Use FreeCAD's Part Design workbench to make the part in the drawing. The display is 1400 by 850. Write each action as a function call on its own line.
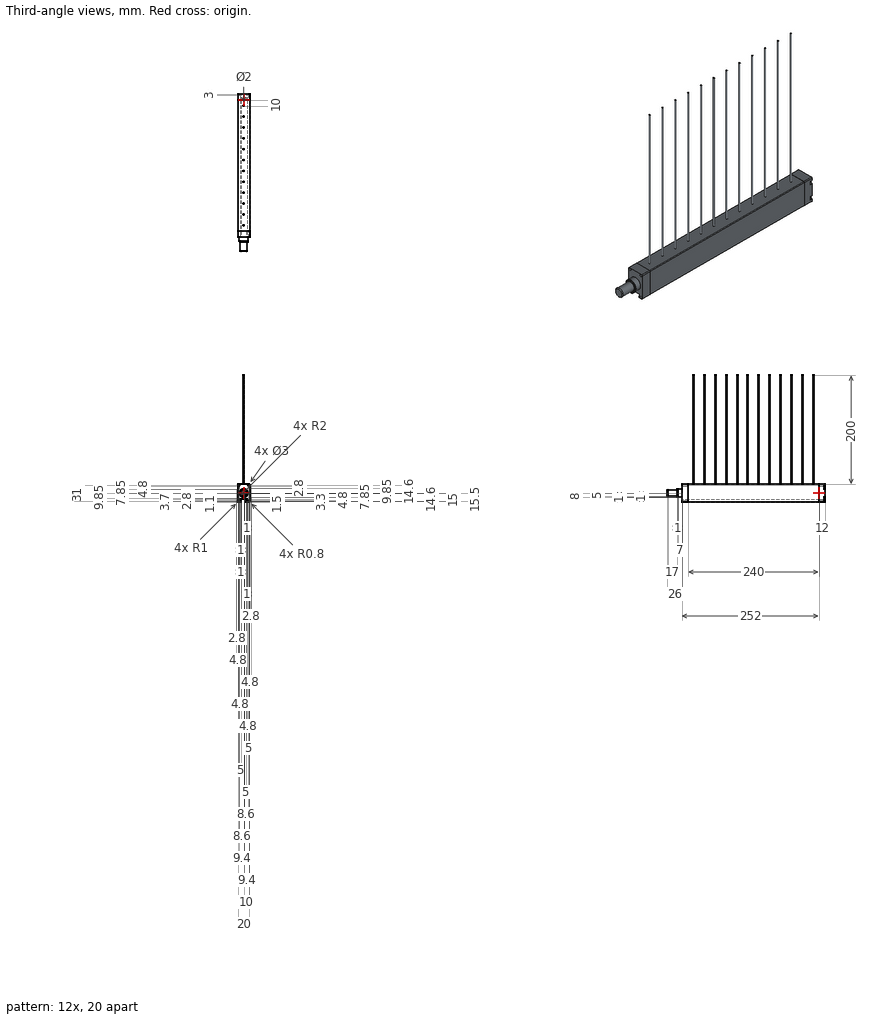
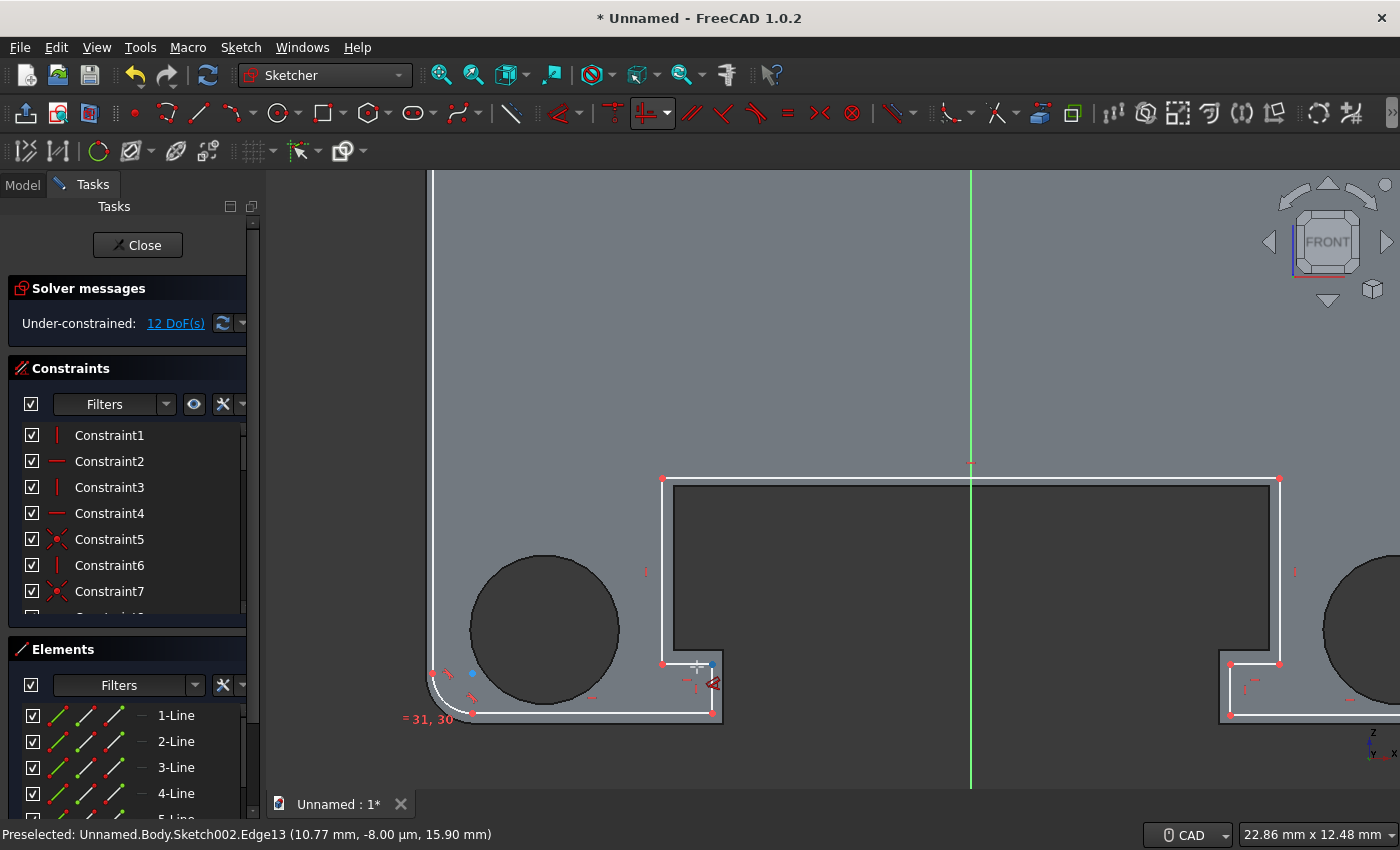
click(697, 664)
click(687, 698)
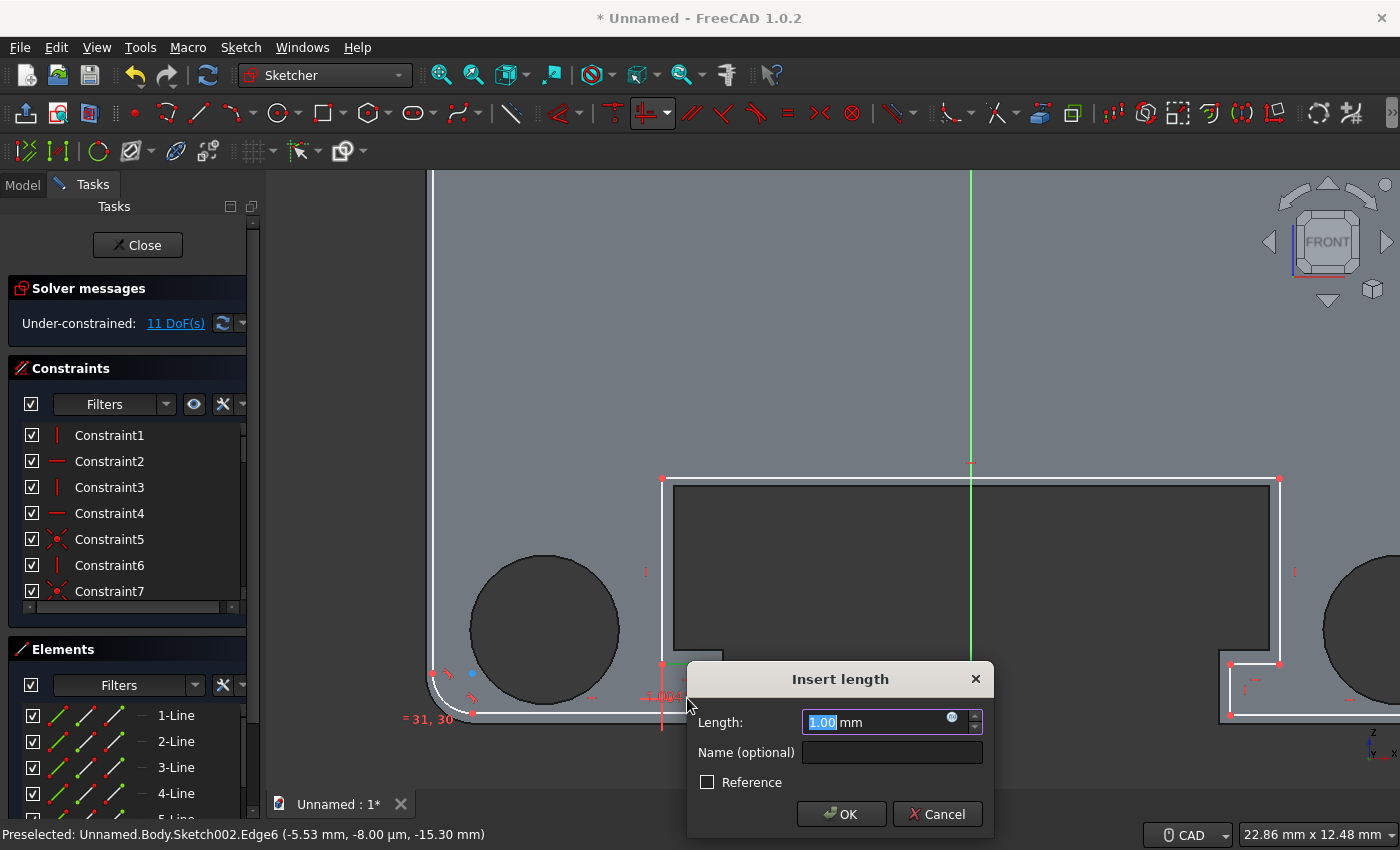
text(1)
key(Return)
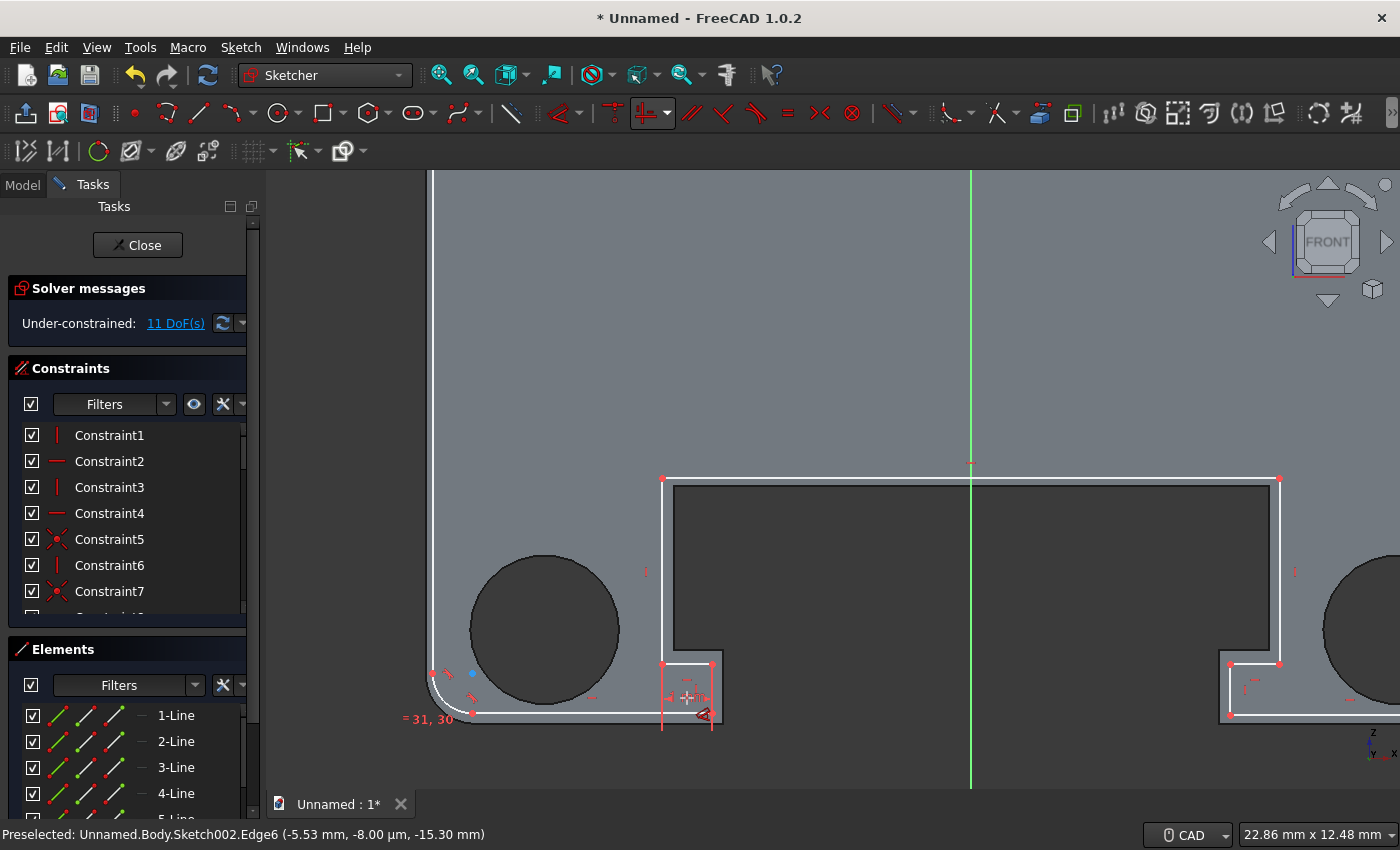
scroll(697, 667, down, 7)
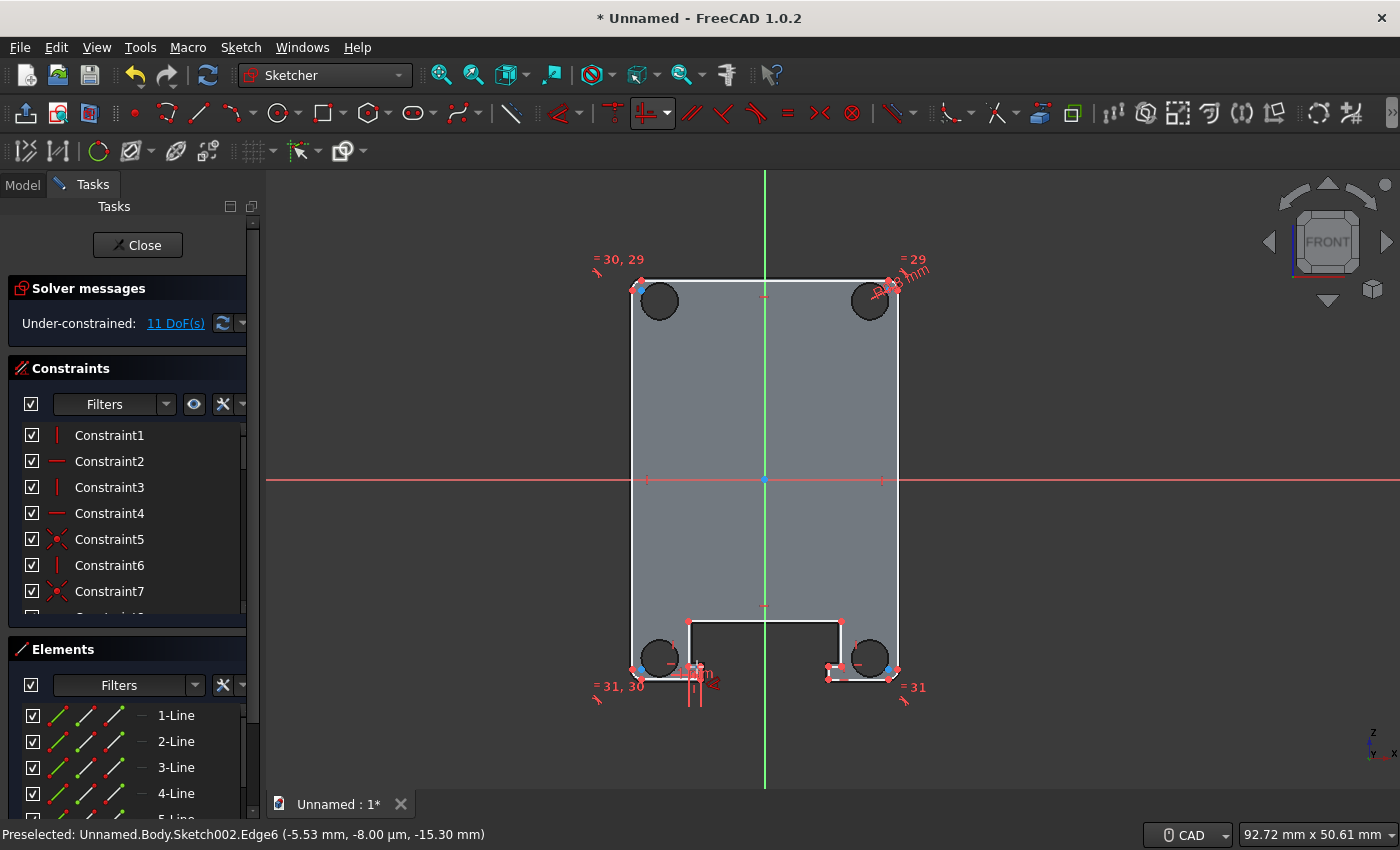
scroll(837, 667, up, 7)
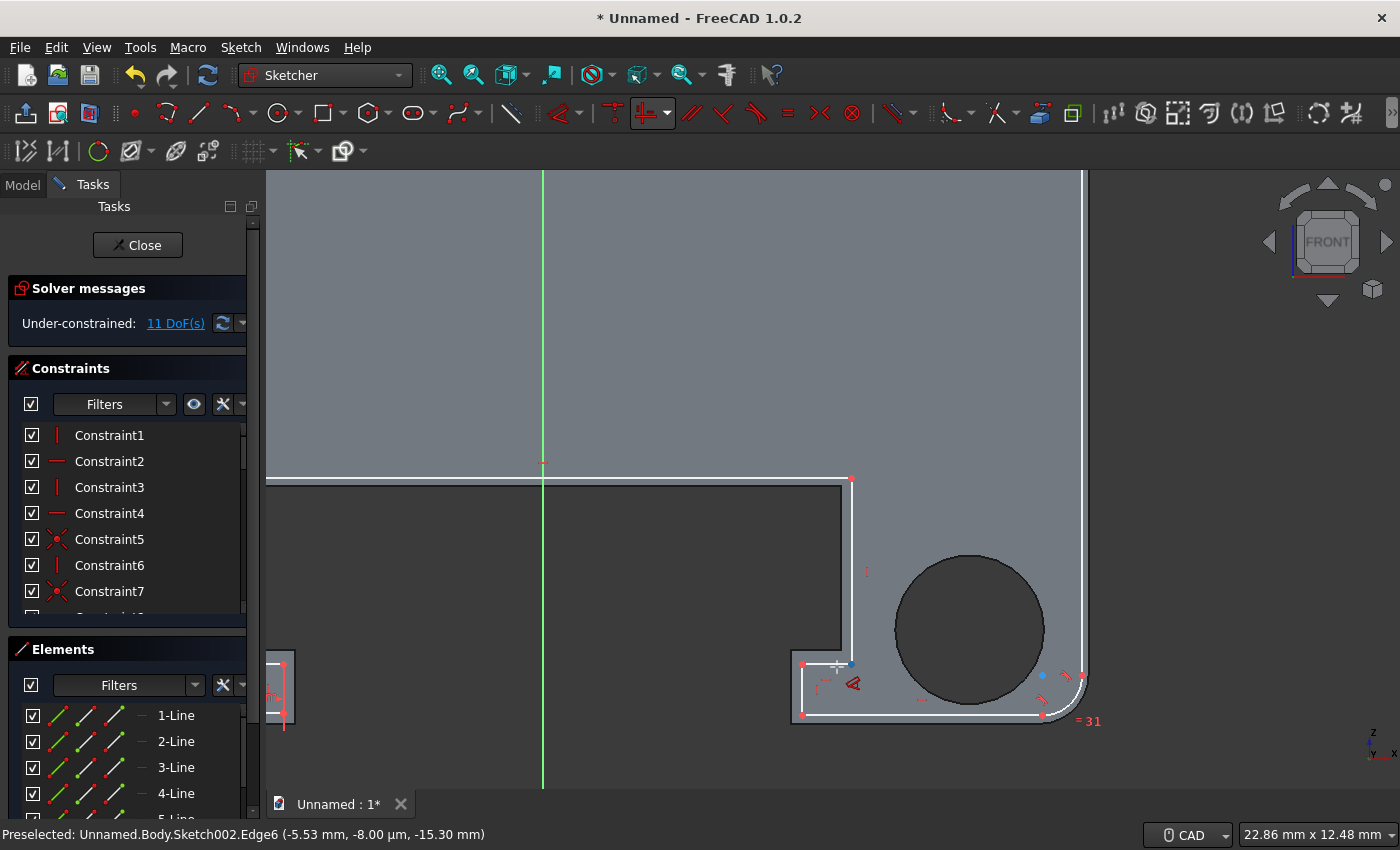
click(837, 664)
click(827, 698)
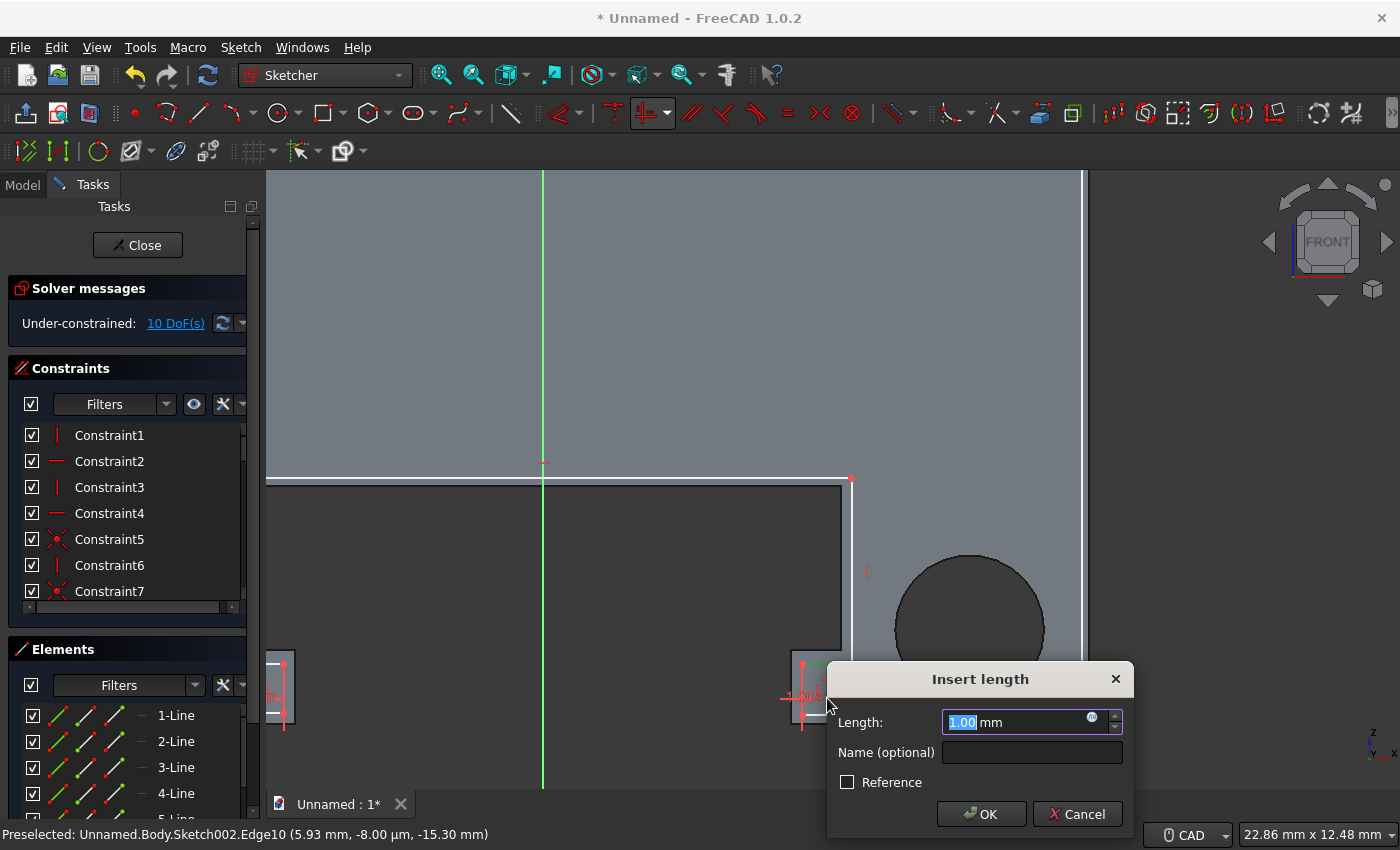
text(1)
key(Return)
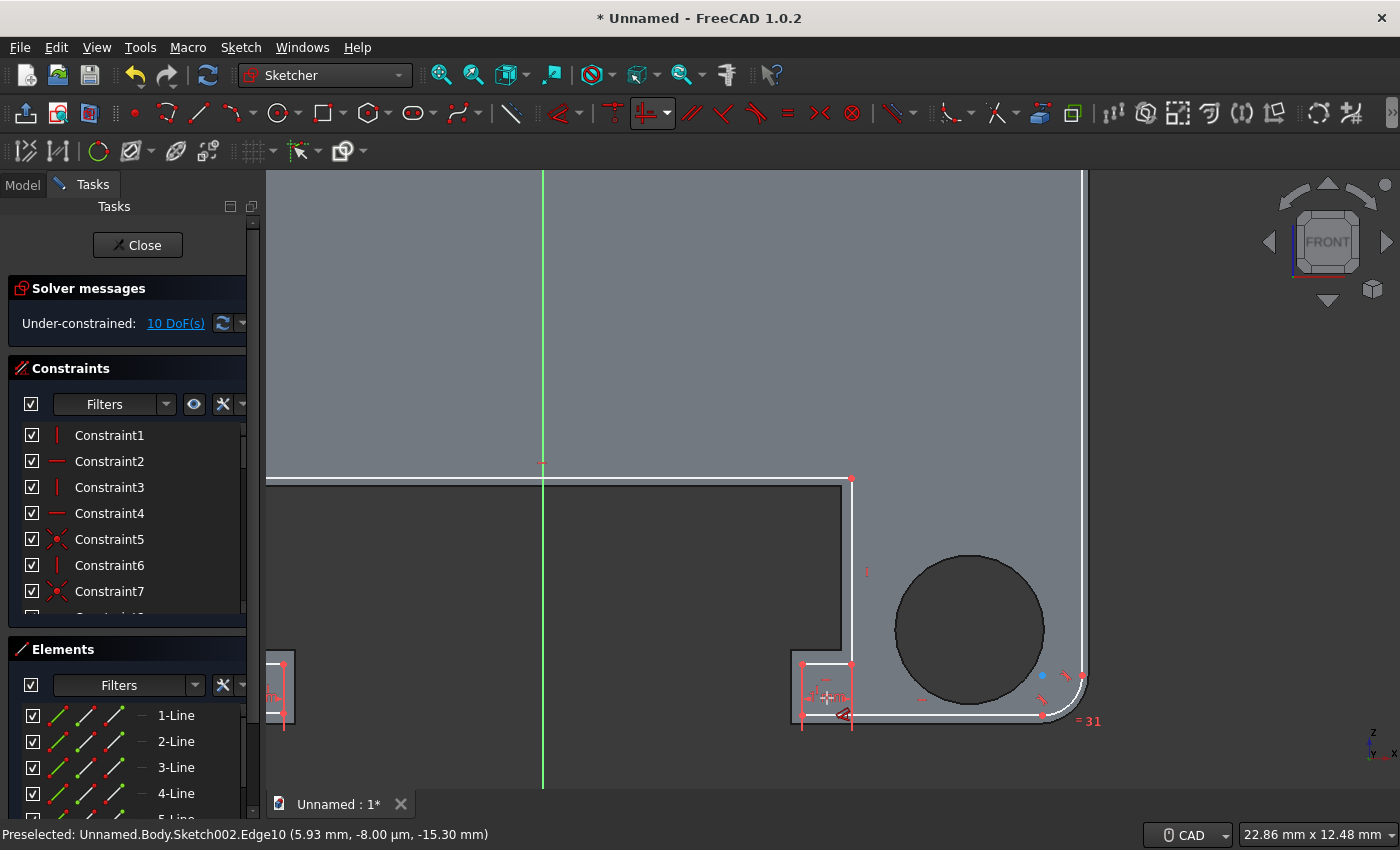
click(1082, 214)
click(1116, 437)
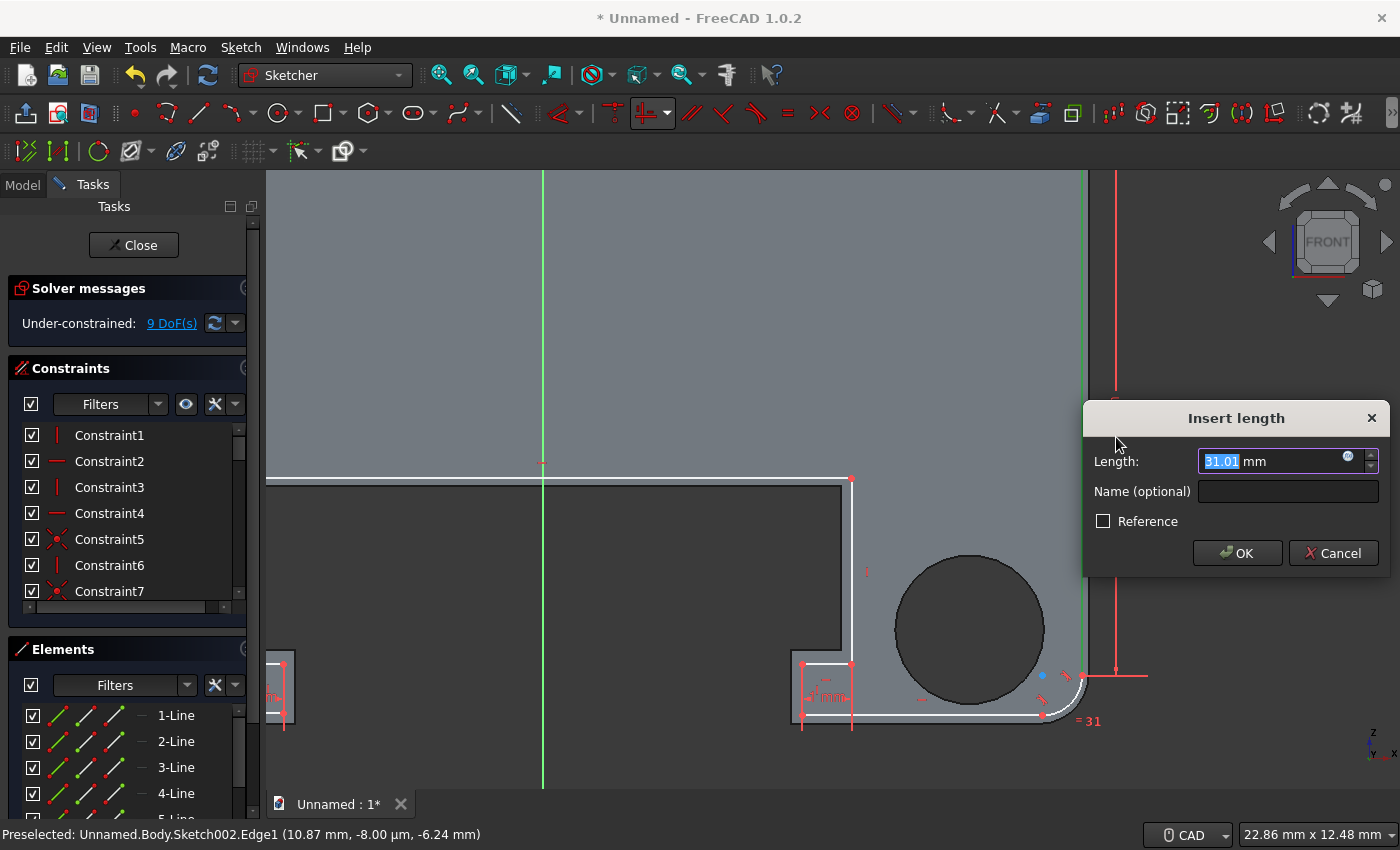
text(31)
key(Return)